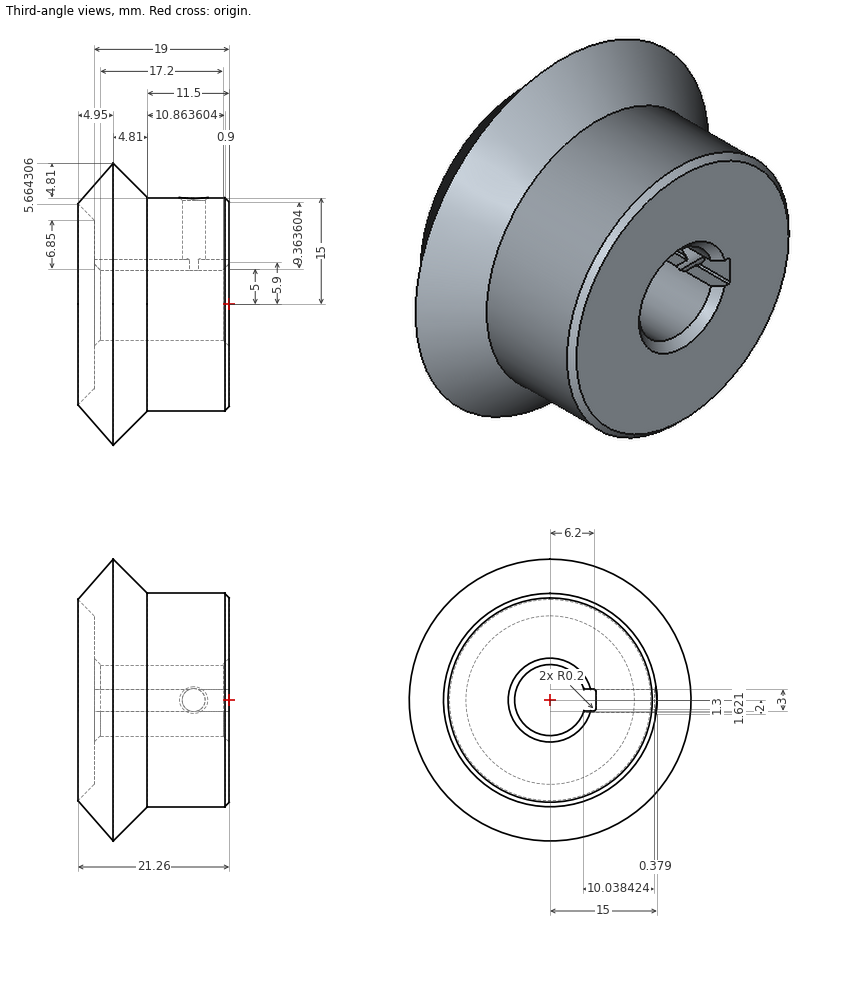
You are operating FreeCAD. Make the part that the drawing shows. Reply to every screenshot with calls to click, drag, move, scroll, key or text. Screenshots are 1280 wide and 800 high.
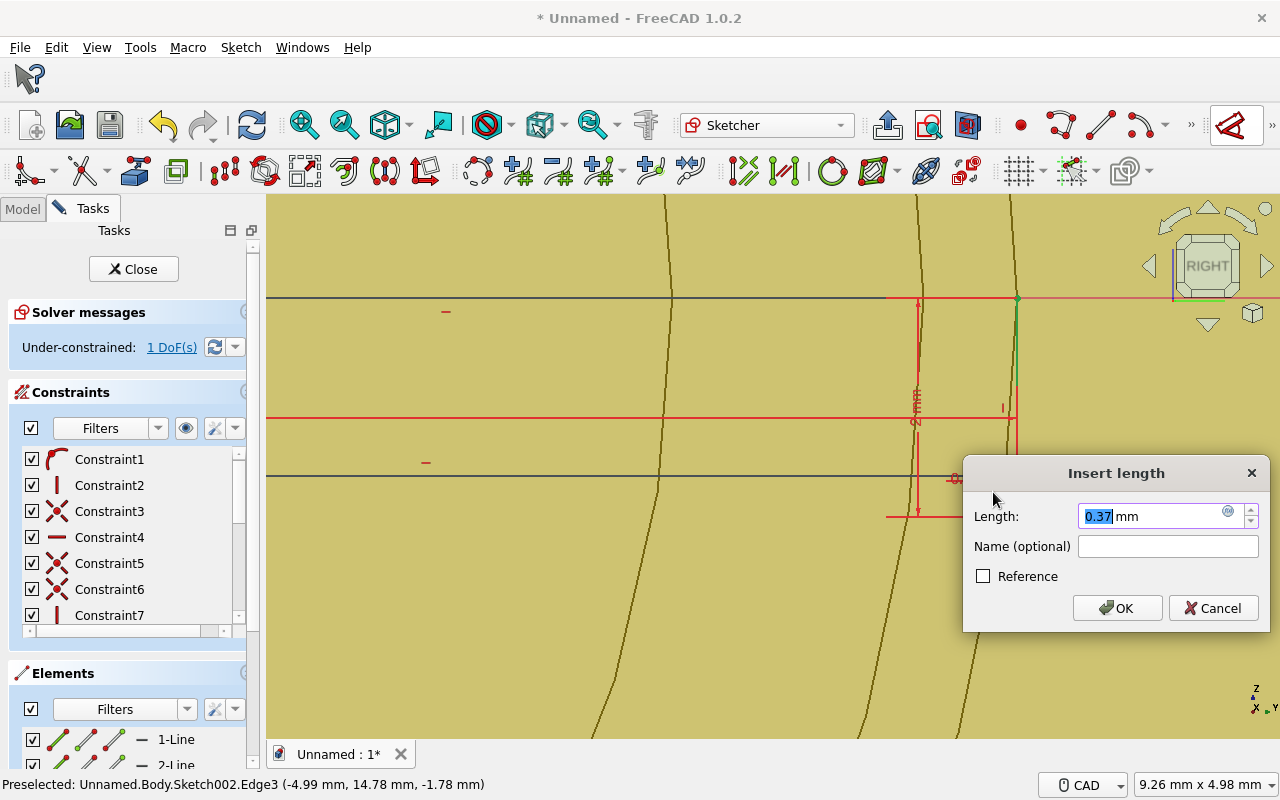
text(0.379)
key(Return)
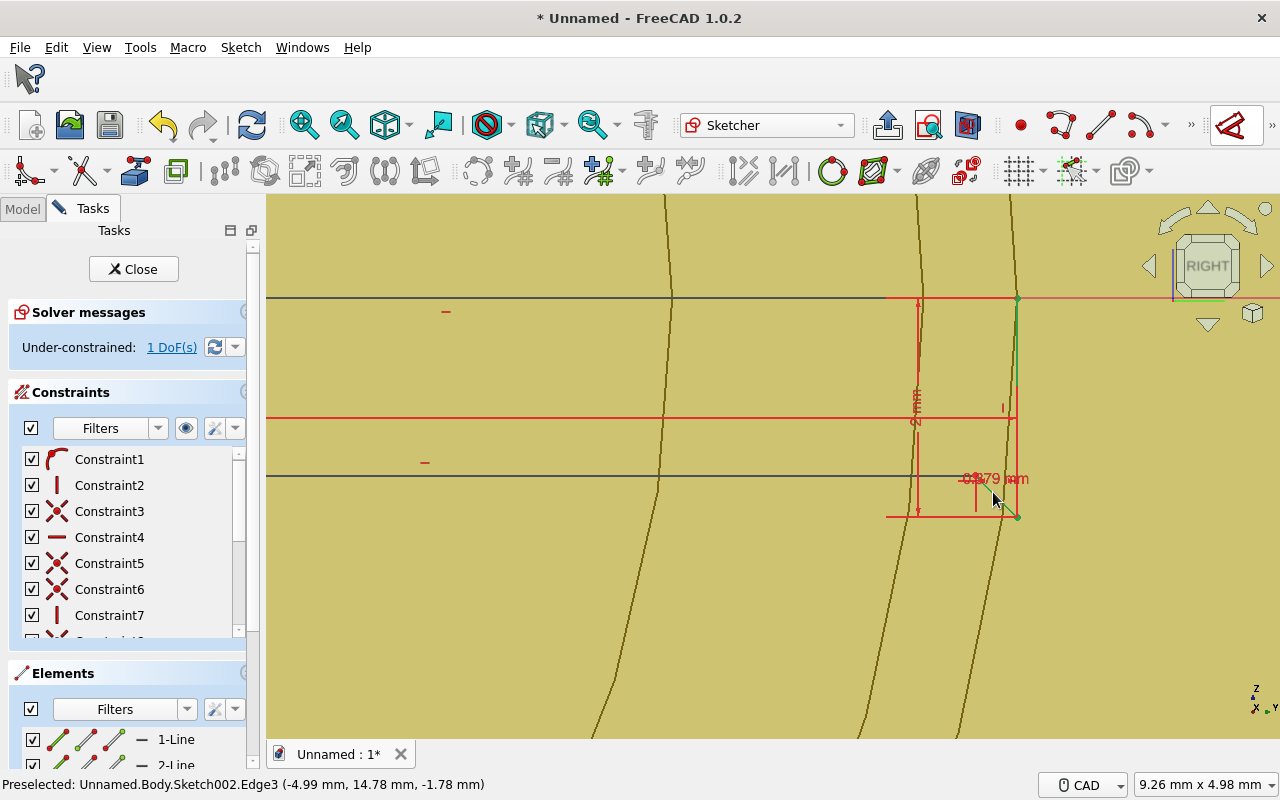
click(646, 476)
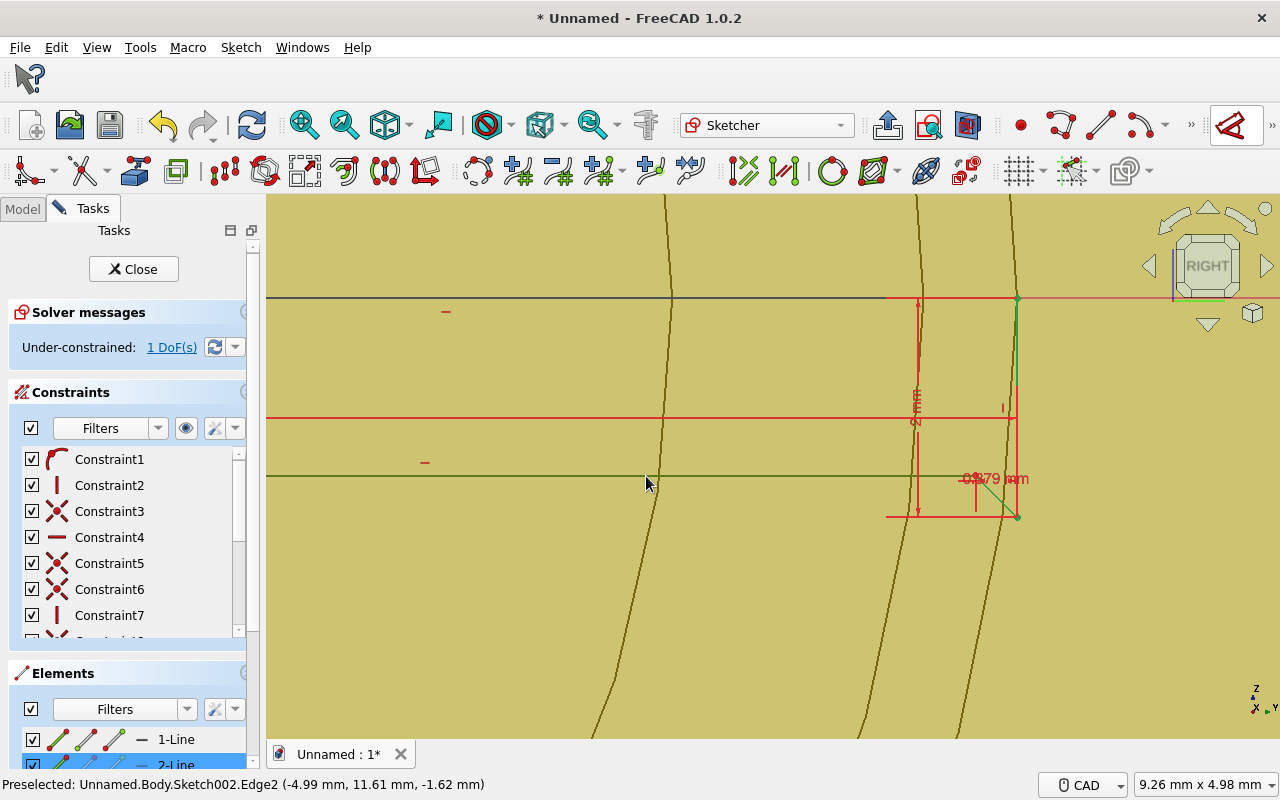
click(1258, 126)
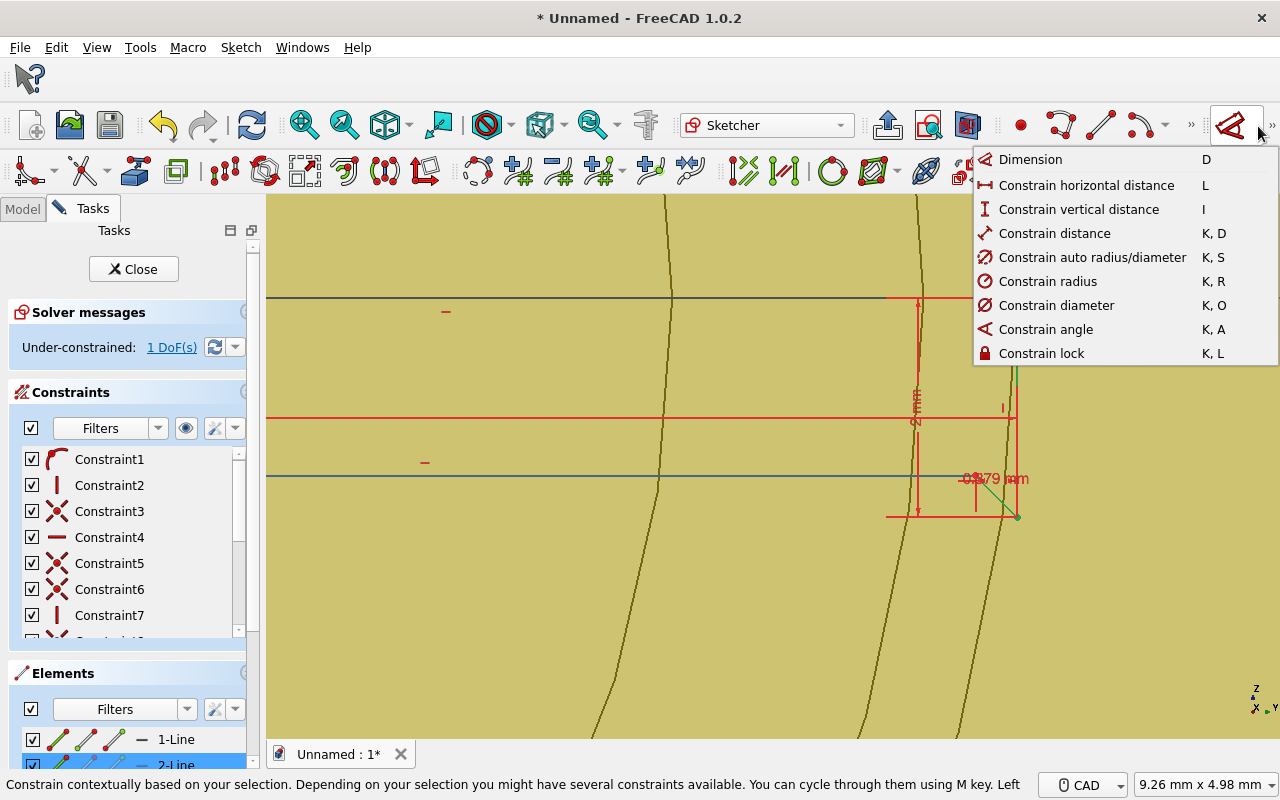
click(1126, 185)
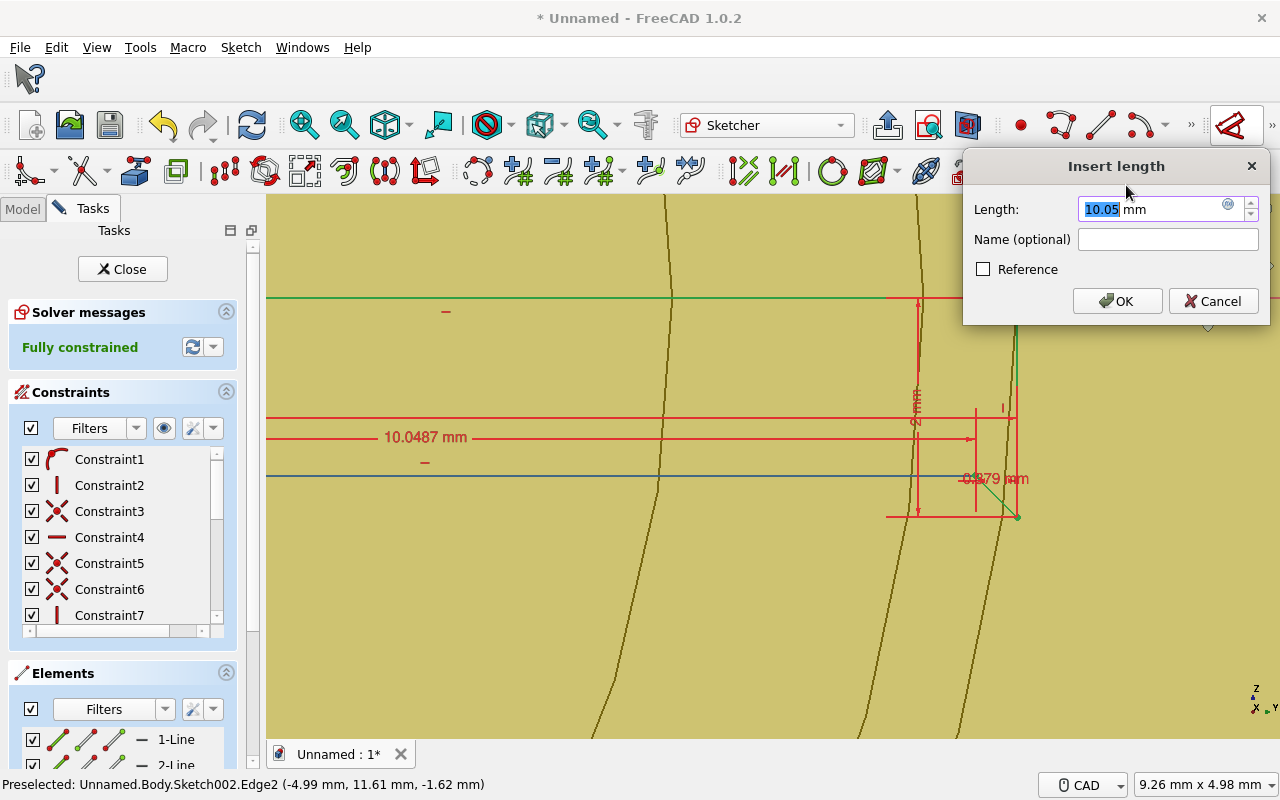
text(10.038424)
key(Return)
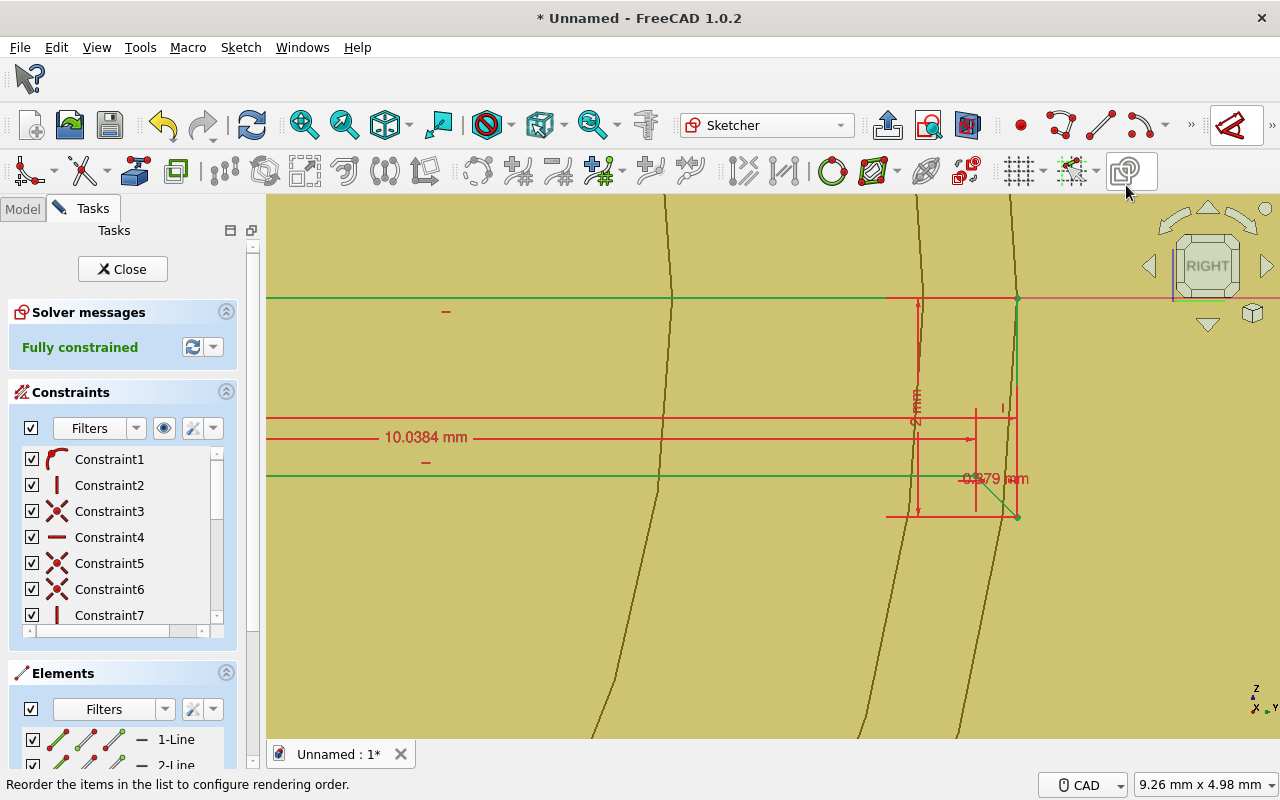
click(123, 269)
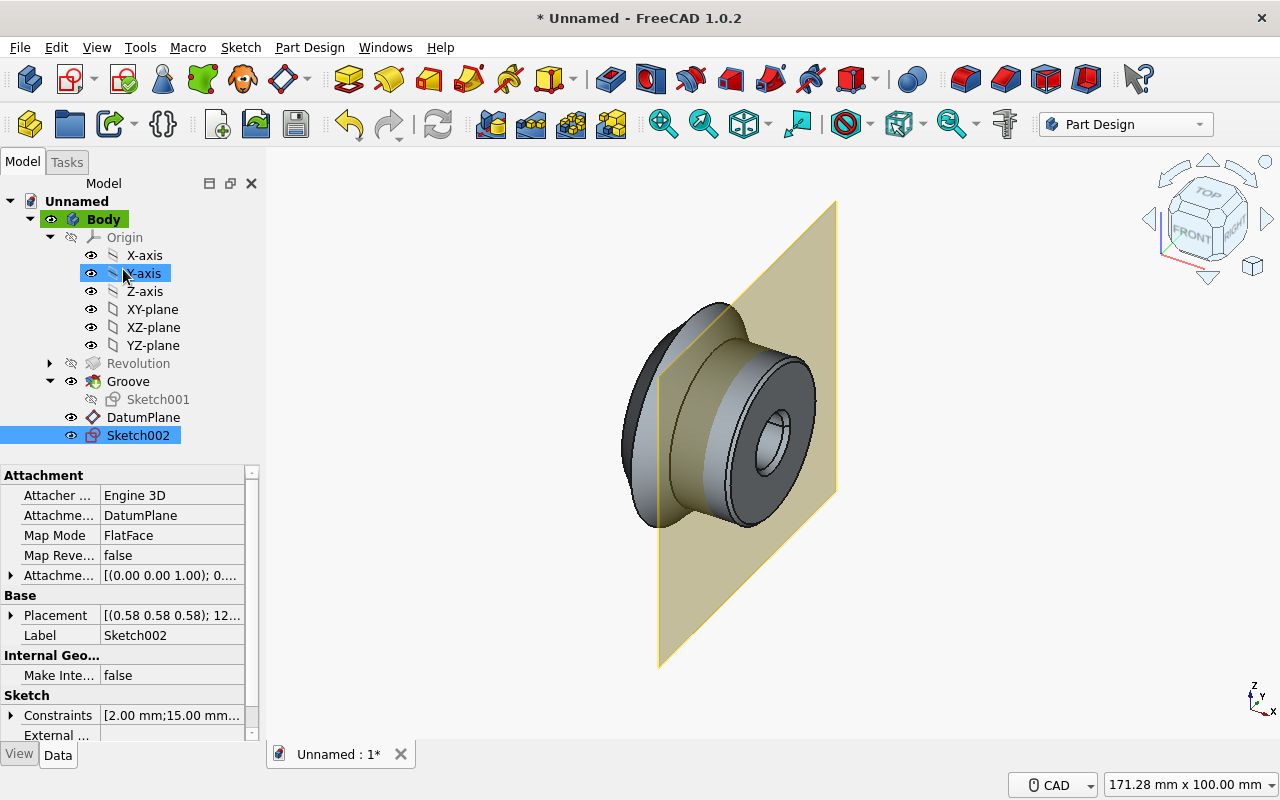
click(692, 80)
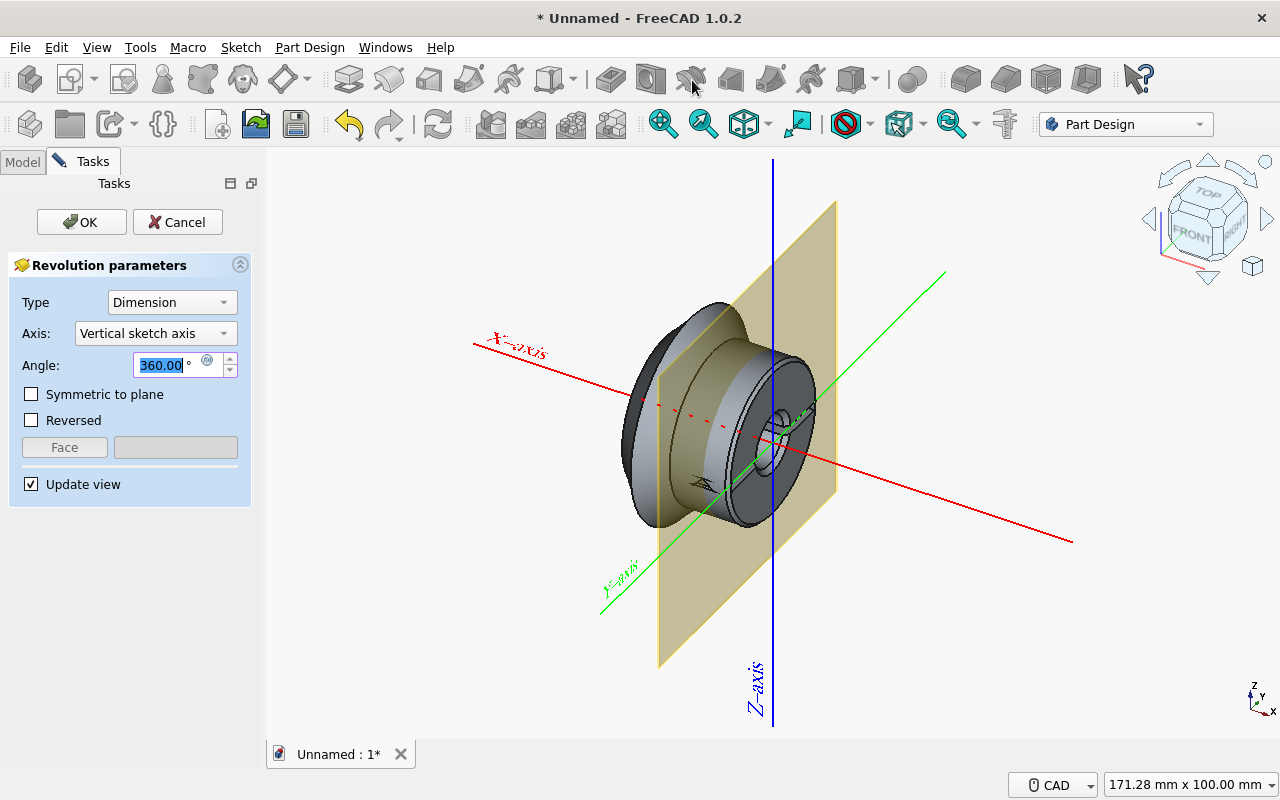
click(156, 334)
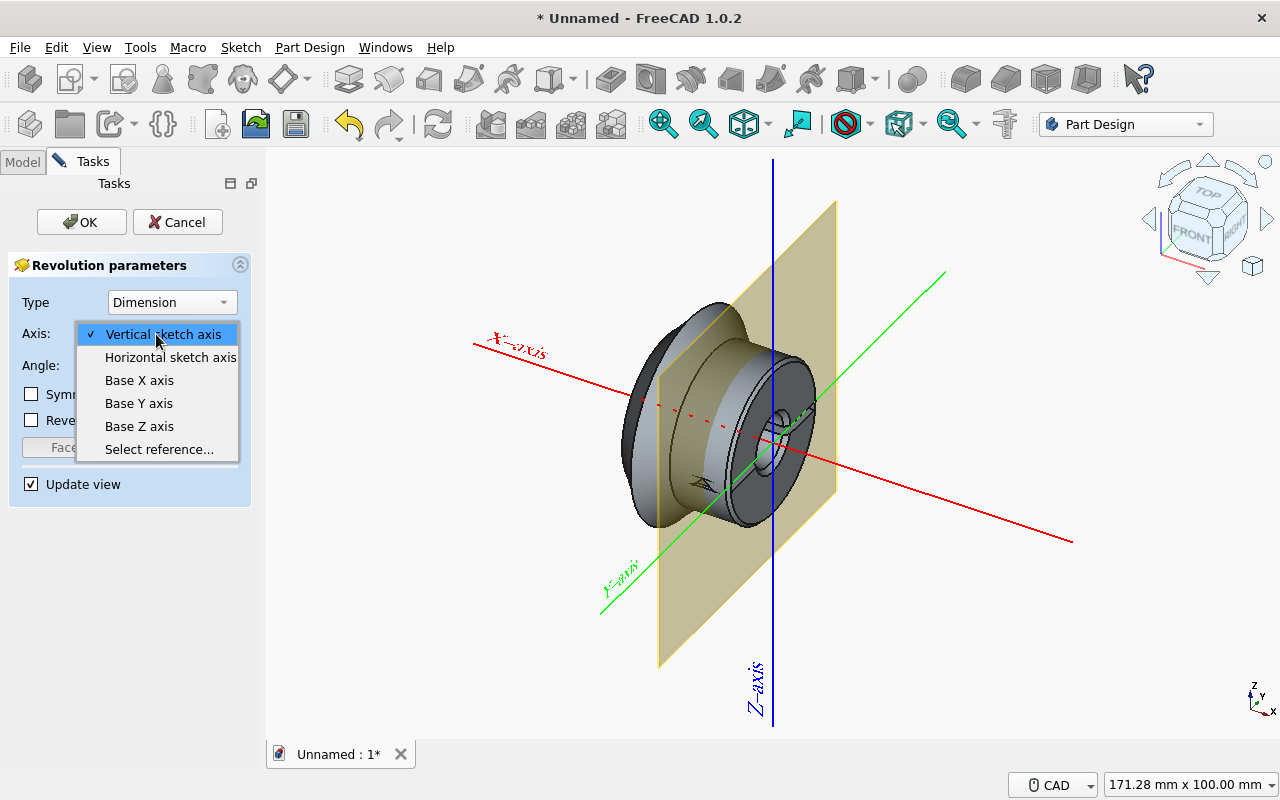
click(156, 358)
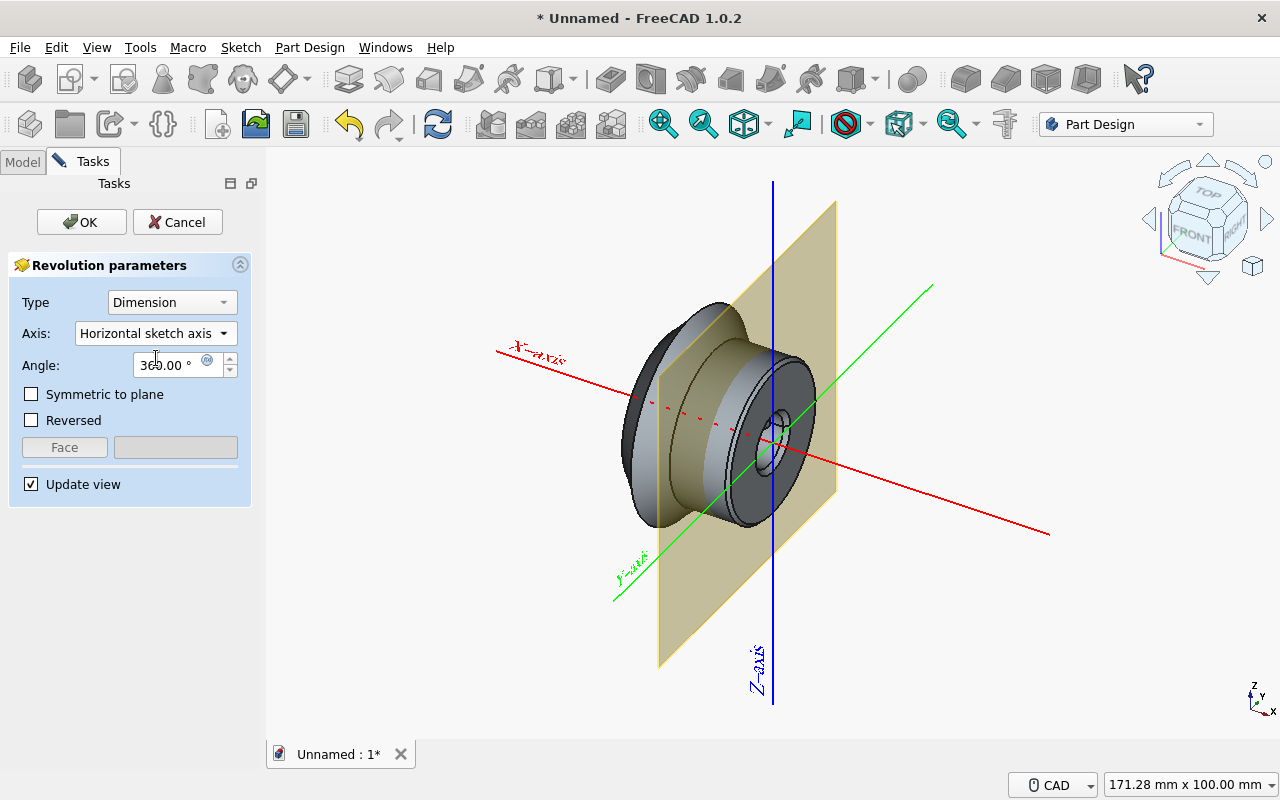
click(82, 222)